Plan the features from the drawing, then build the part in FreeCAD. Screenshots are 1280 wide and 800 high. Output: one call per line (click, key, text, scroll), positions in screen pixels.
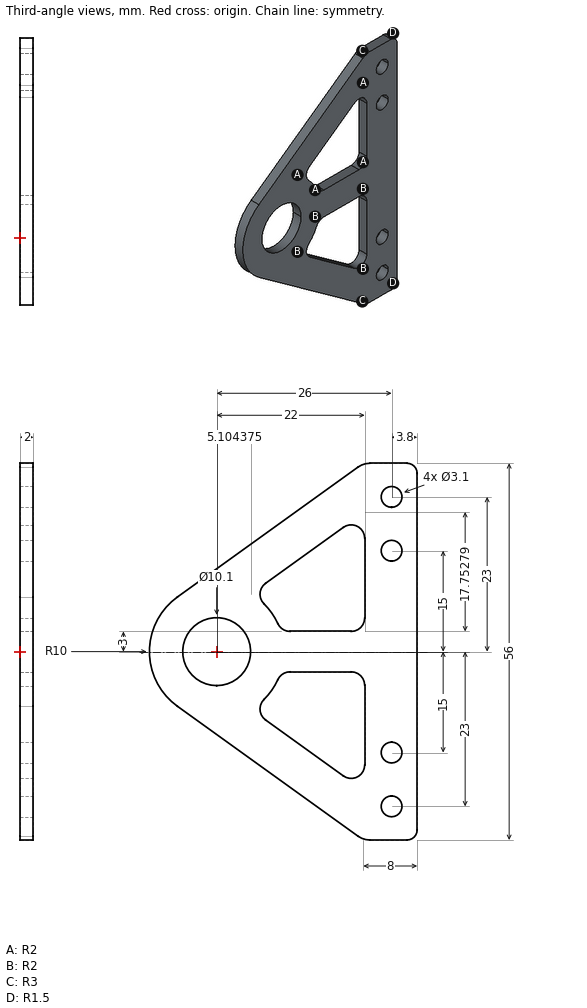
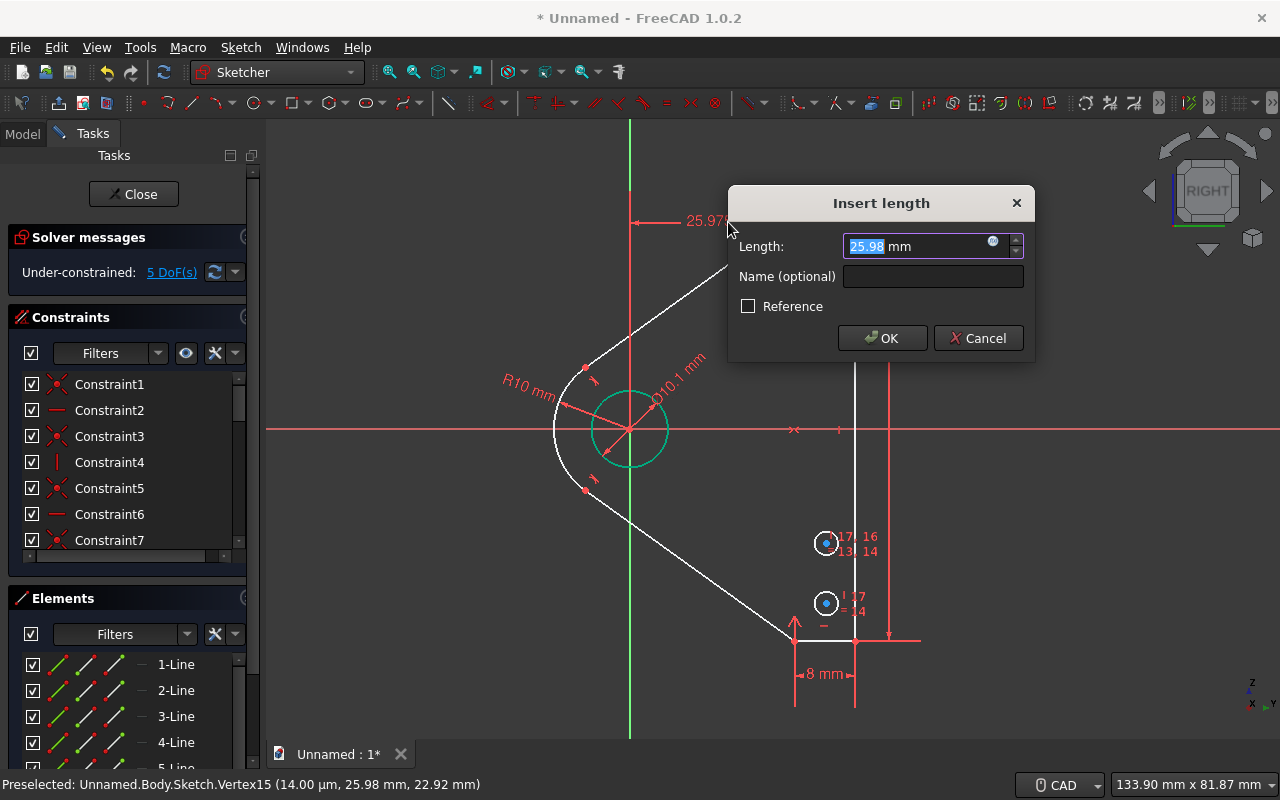
text(26)
key(Return)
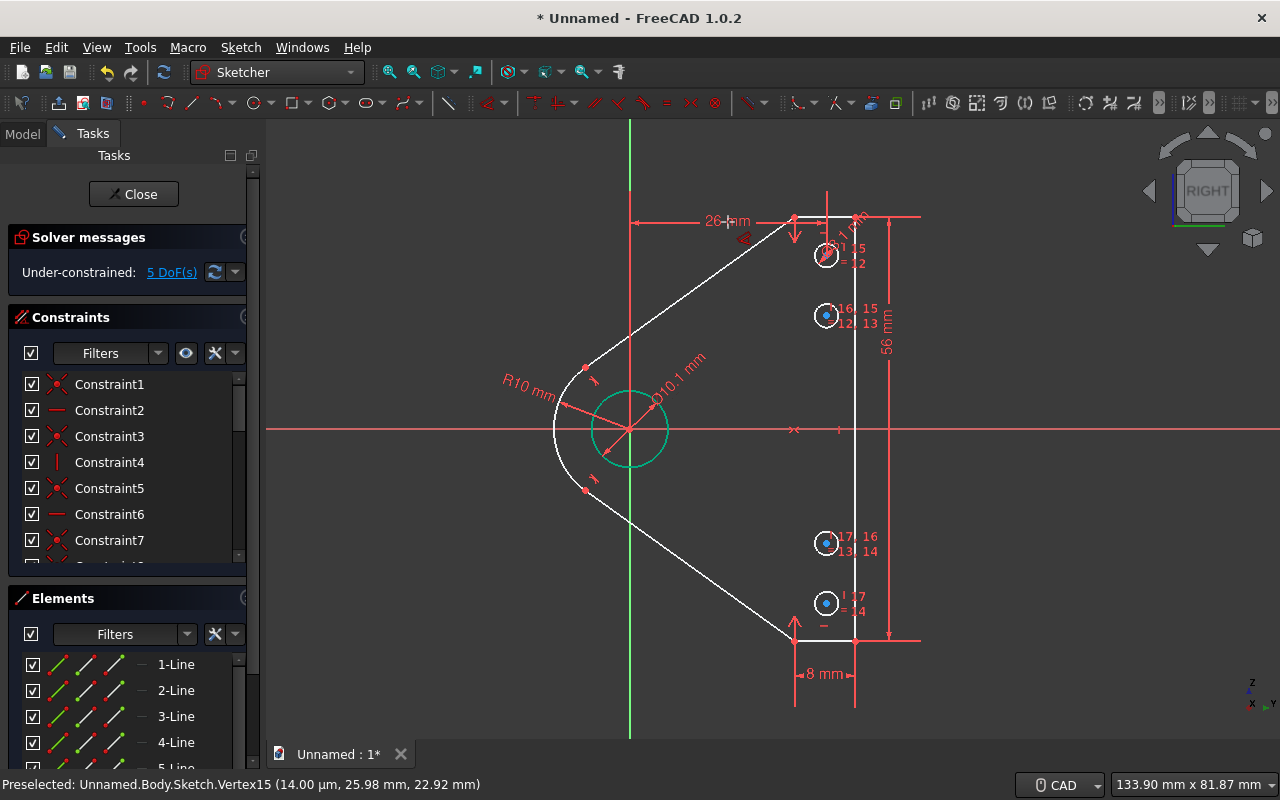
click(827, 256)
click(596, 342)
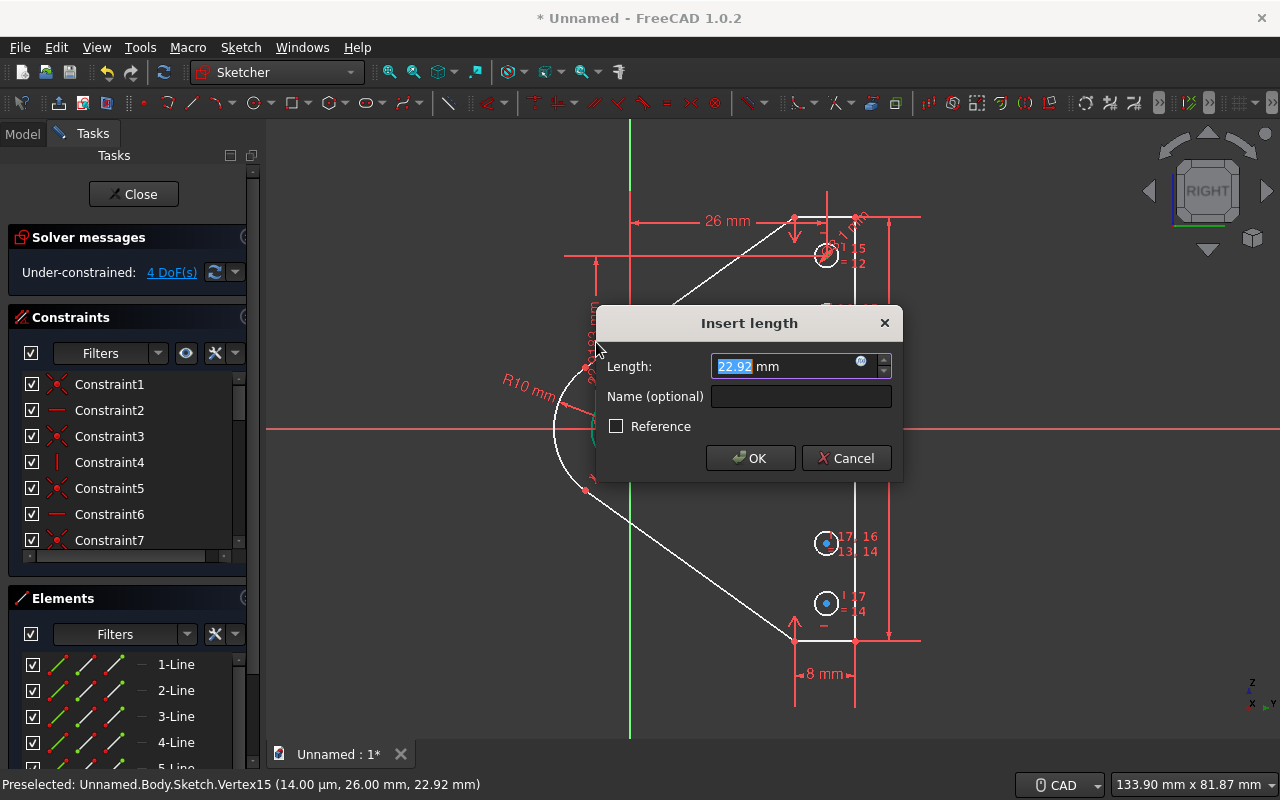
text(23)
key(Return)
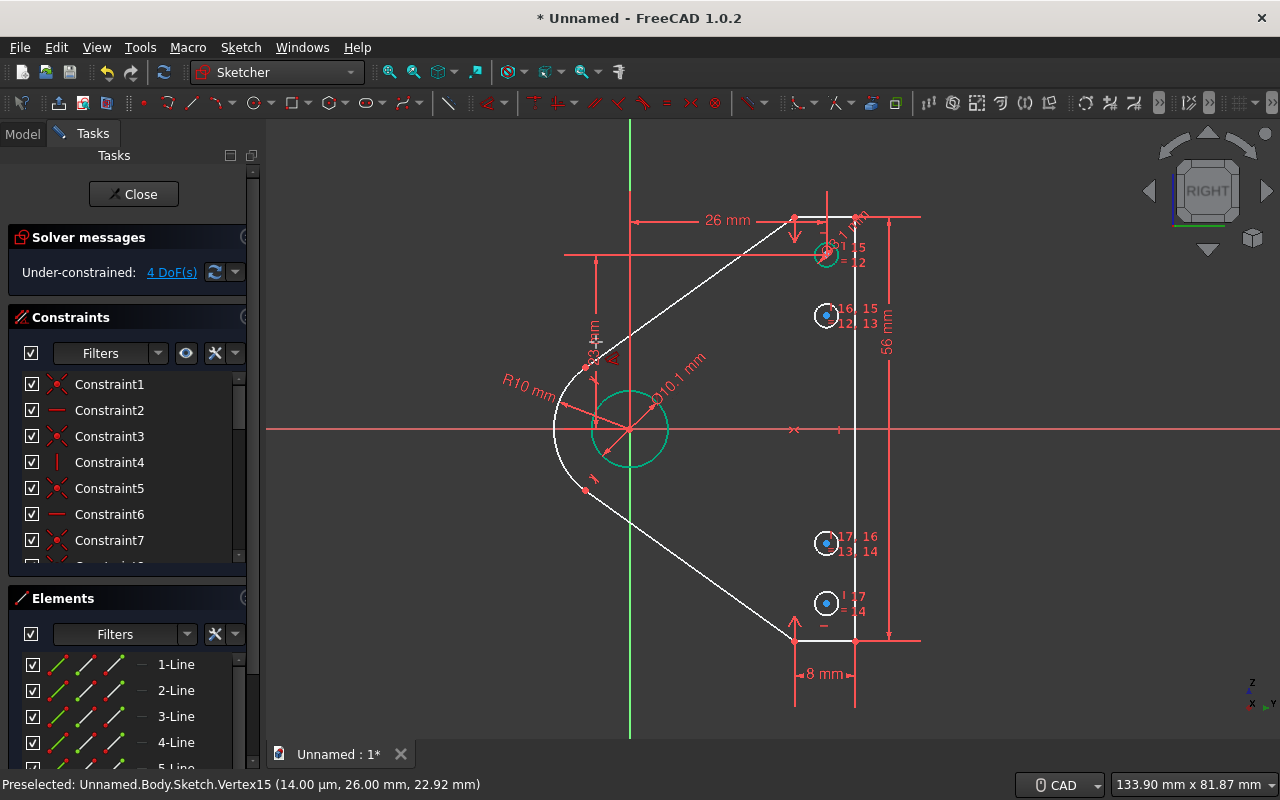
click(827, 316)
click(885, 372)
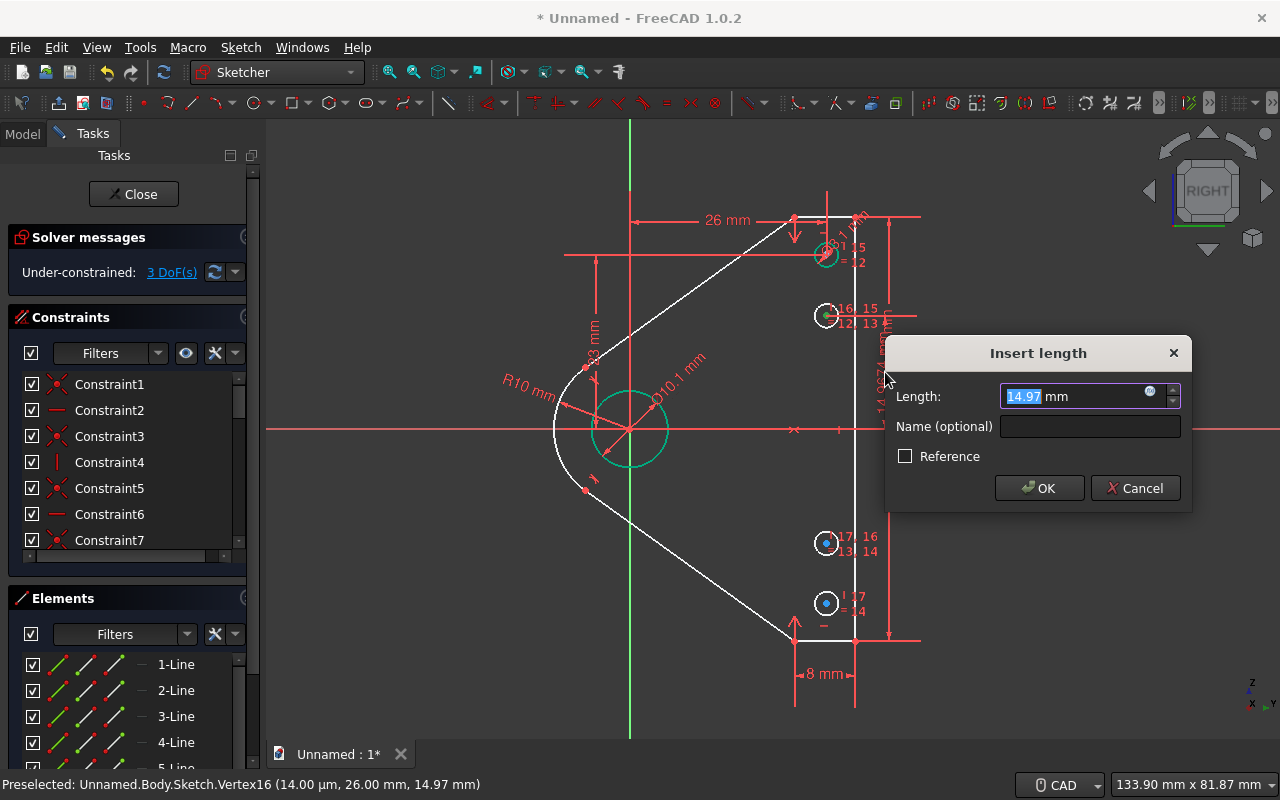
text(15)
key(Return)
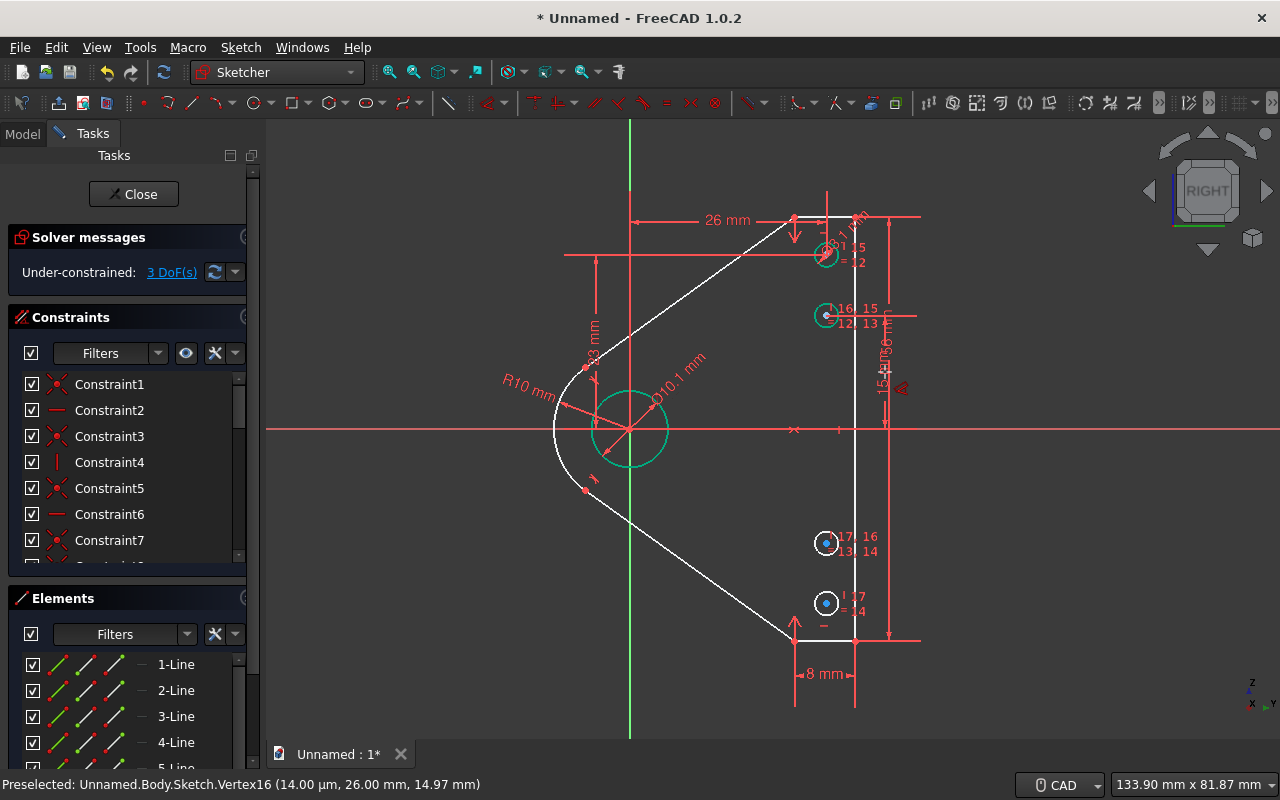
click(827, 543)
click(596, 526)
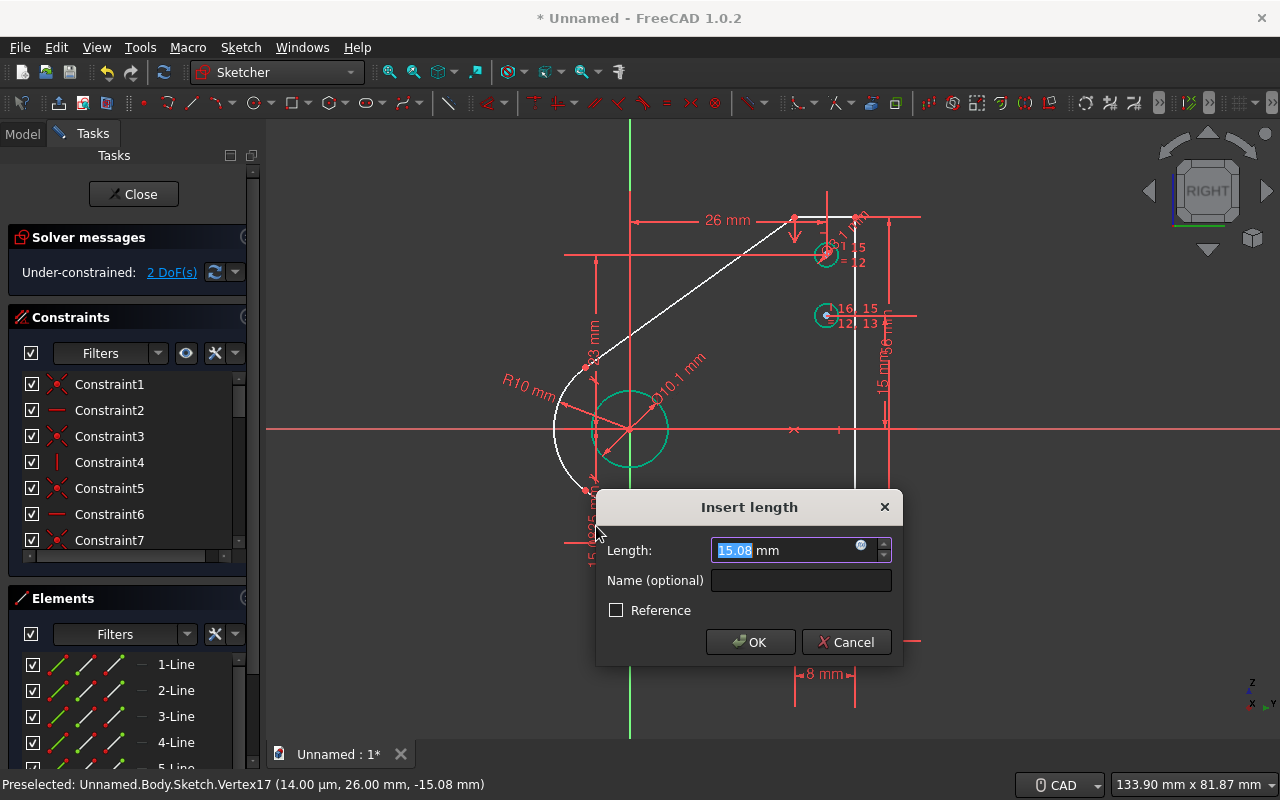
text(15)
key(Return)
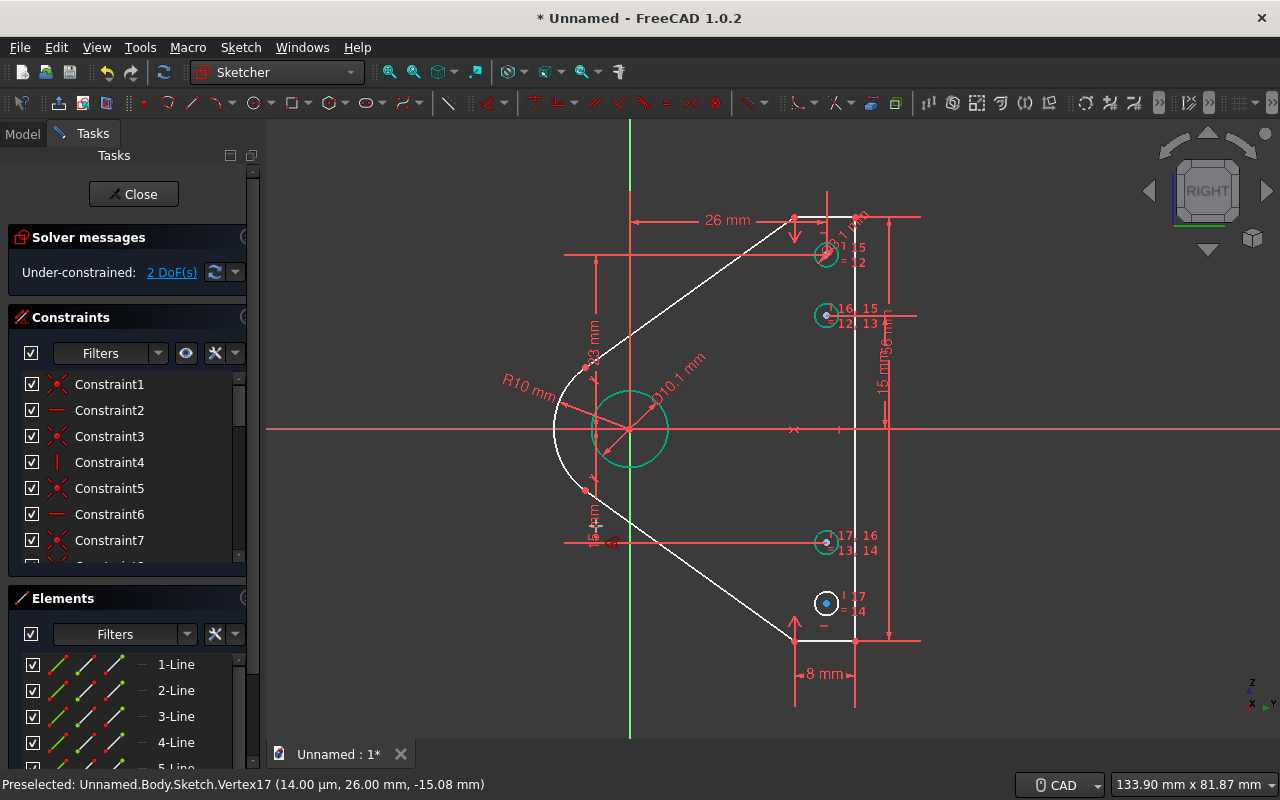
click(827, 604)
click(596, 476)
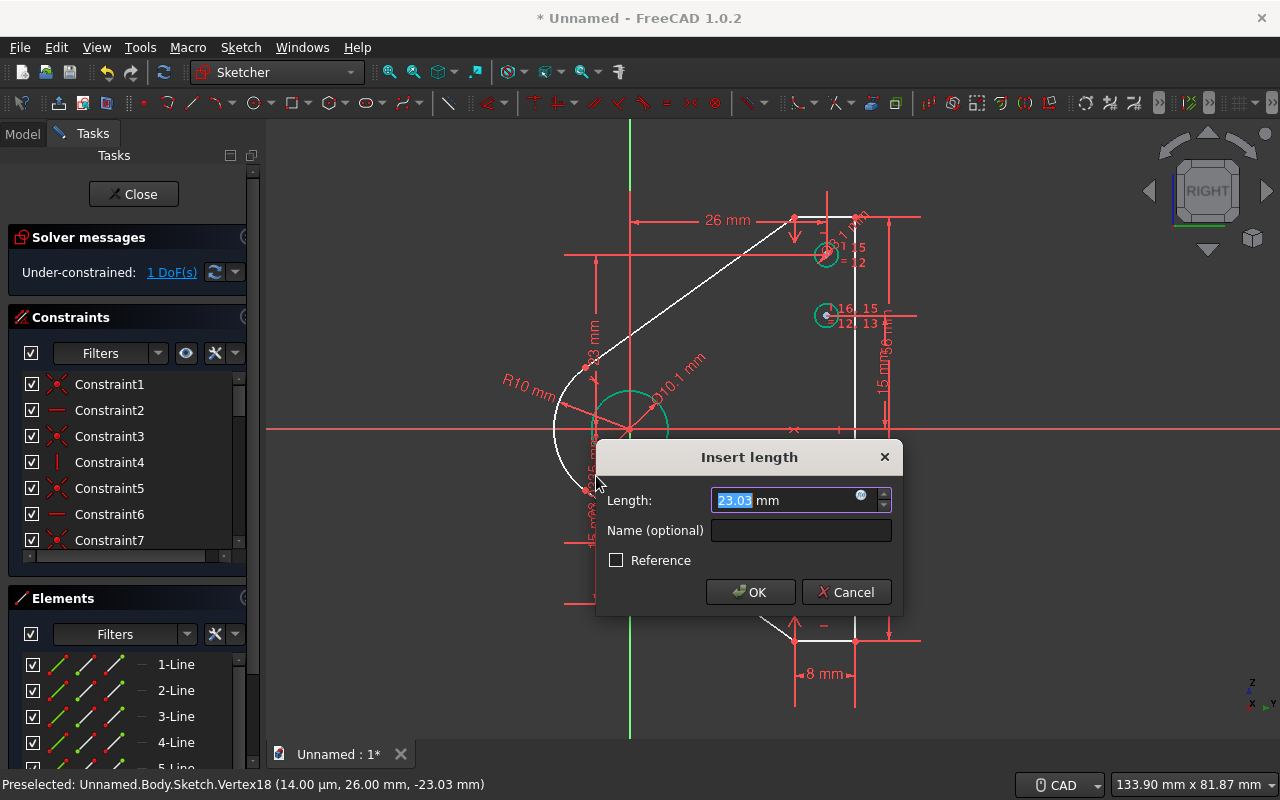
text(23)
key(Return)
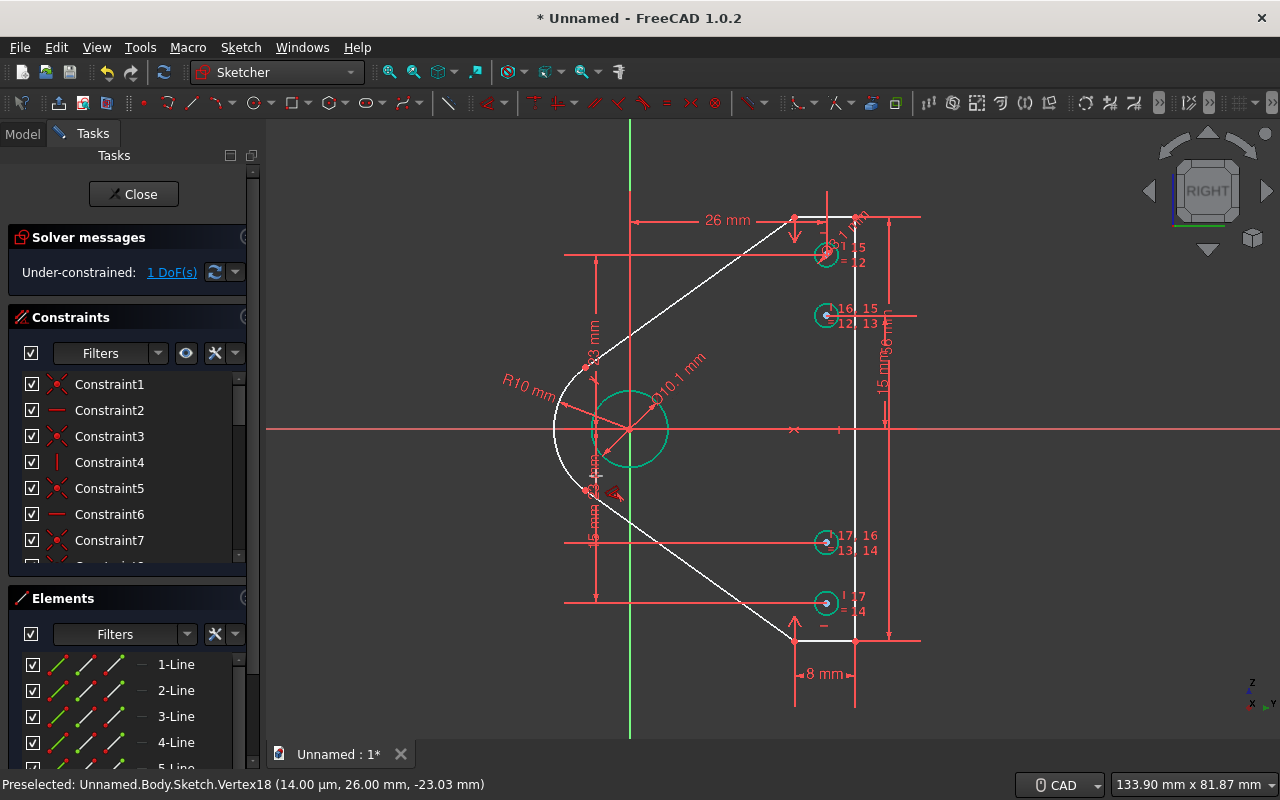
scroll(855, 217, up, 2)